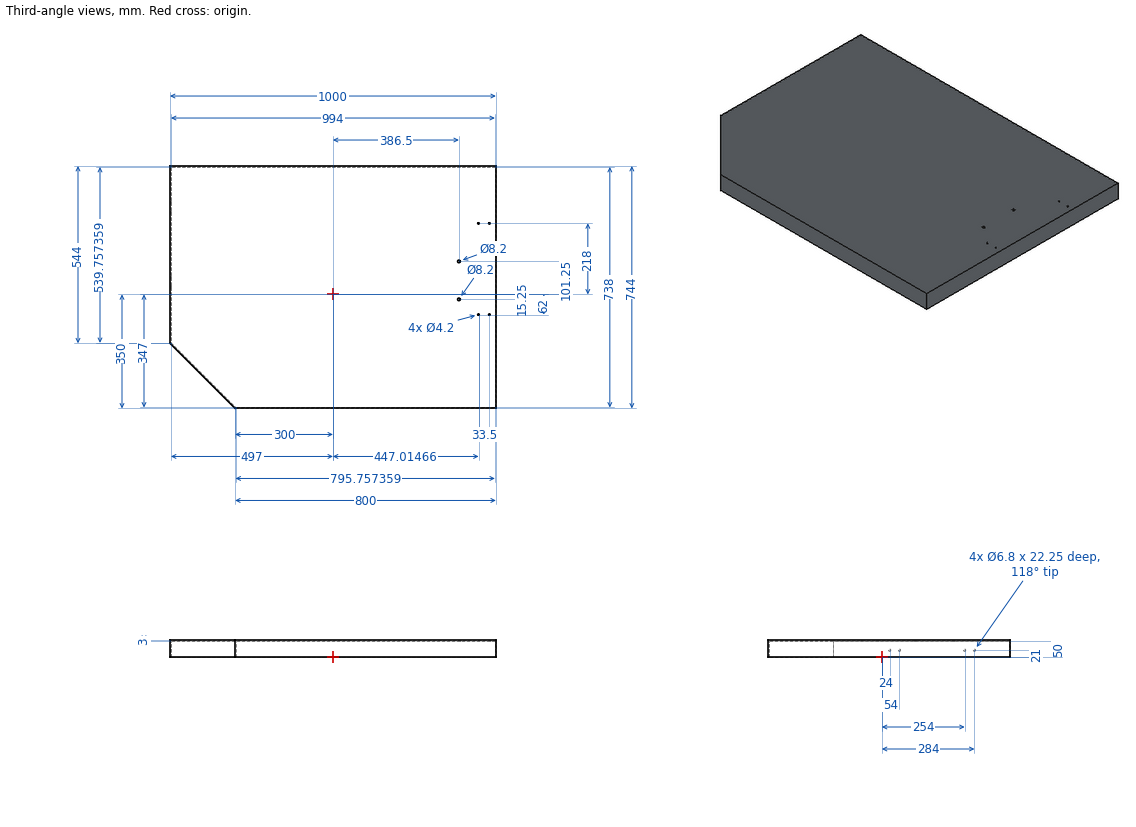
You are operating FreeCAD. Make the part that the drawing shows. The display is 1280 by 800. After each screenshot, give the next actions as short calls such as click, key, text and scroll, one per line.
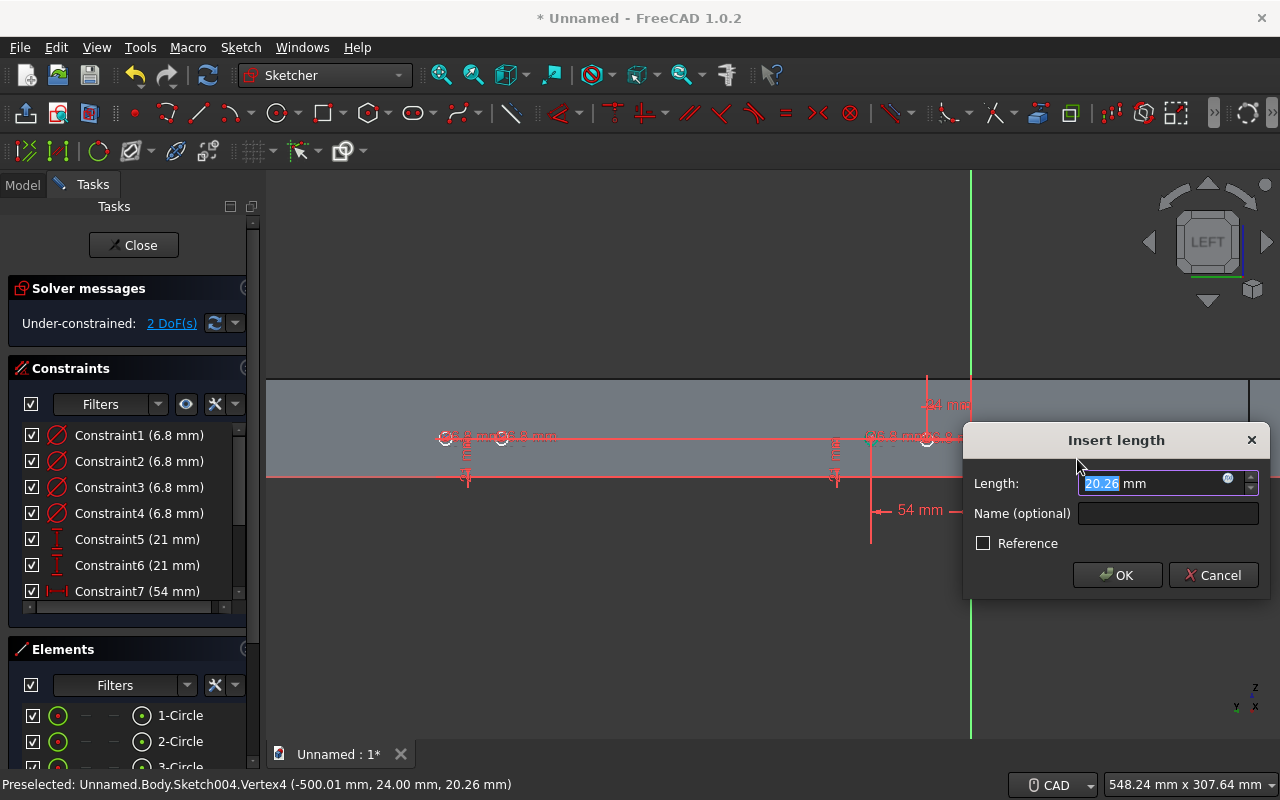
text(21)
key(Return)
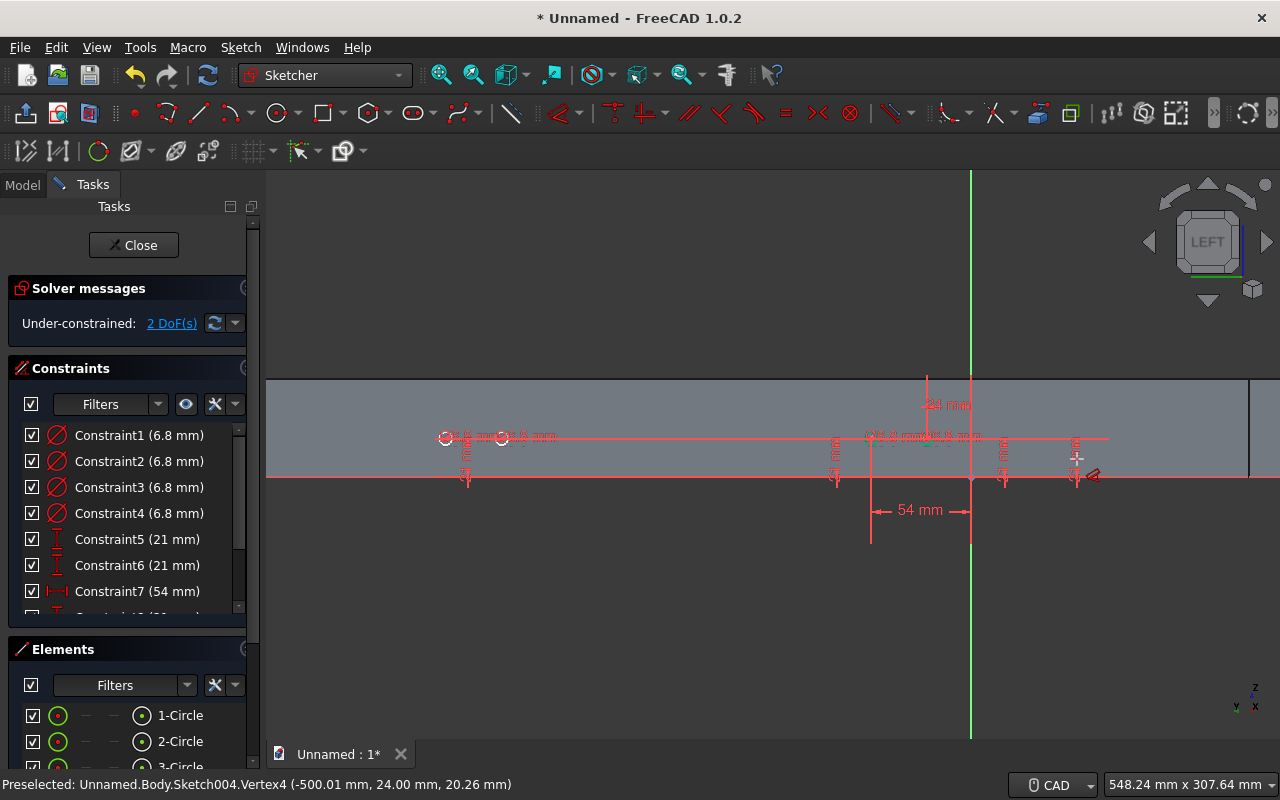
click(446, 439)
click(708, 511)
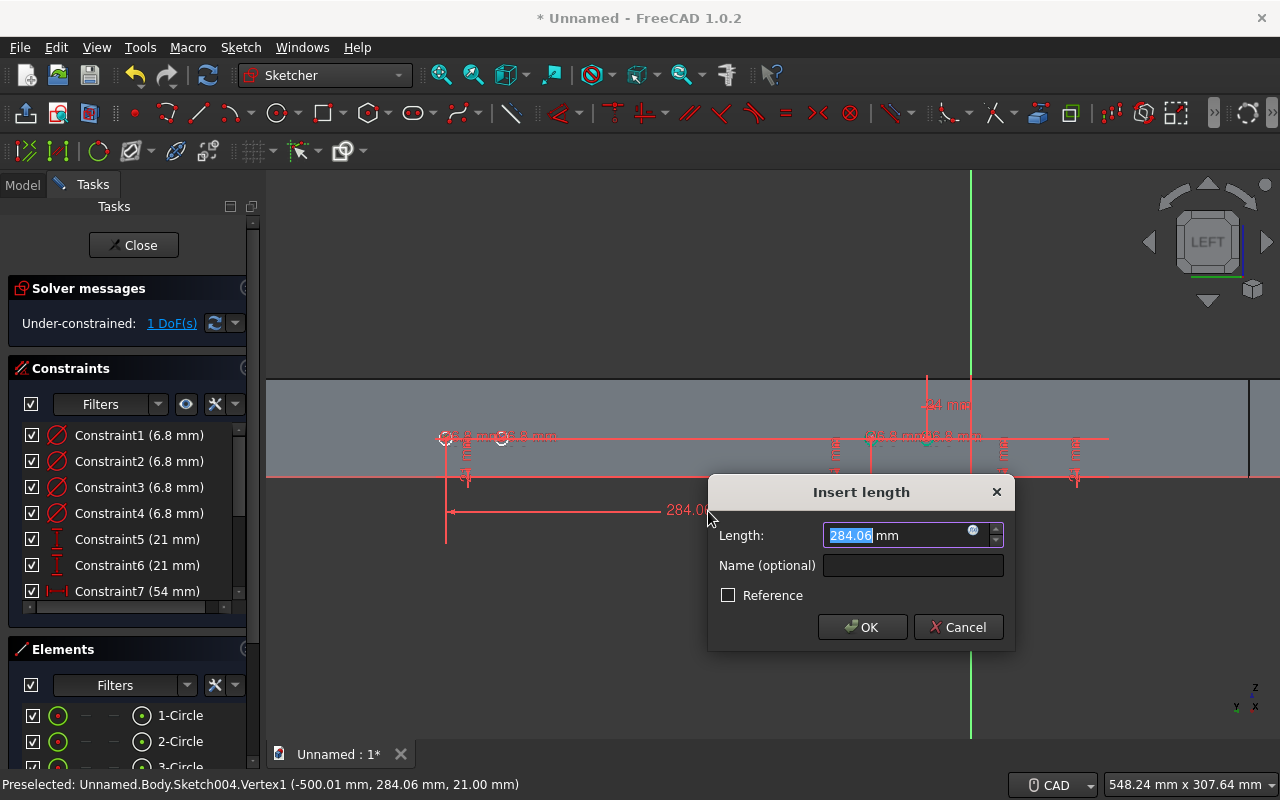
text(284)
key(Return)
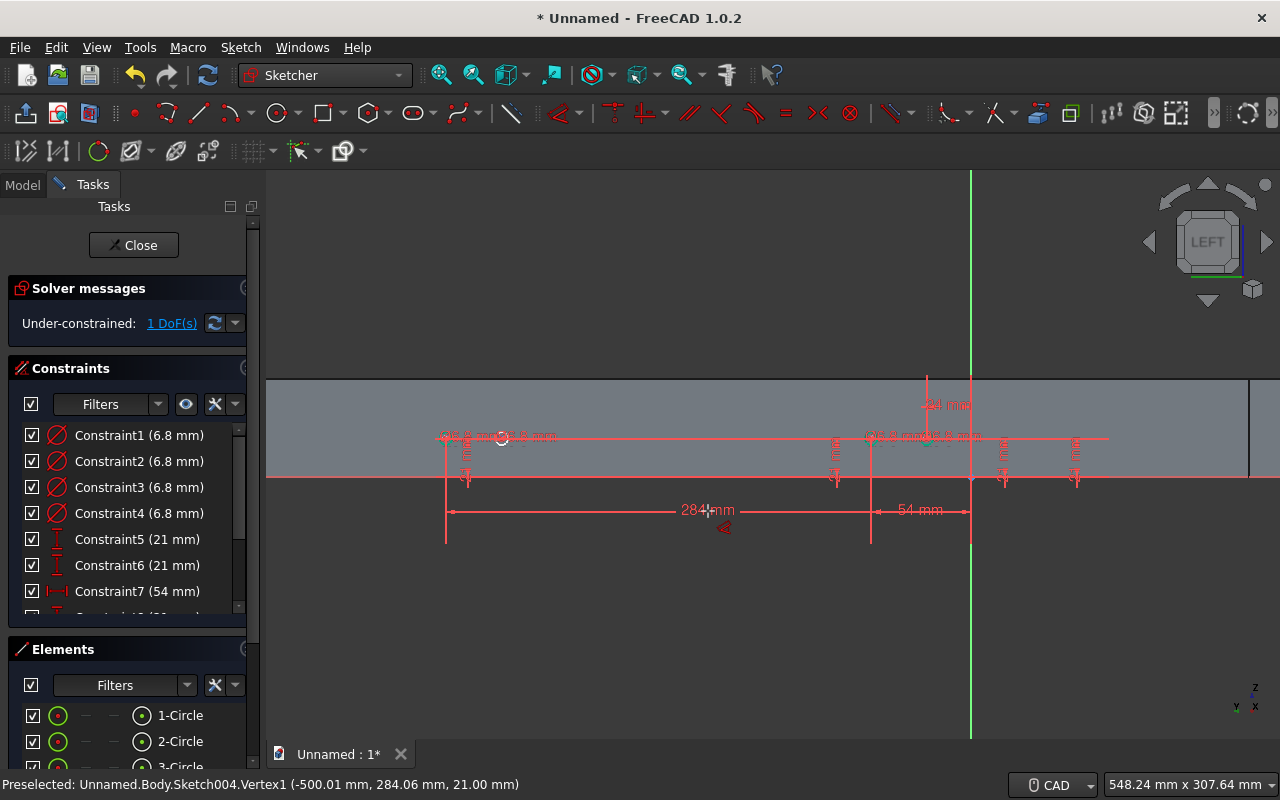
click(502, 439)
click(628, 511)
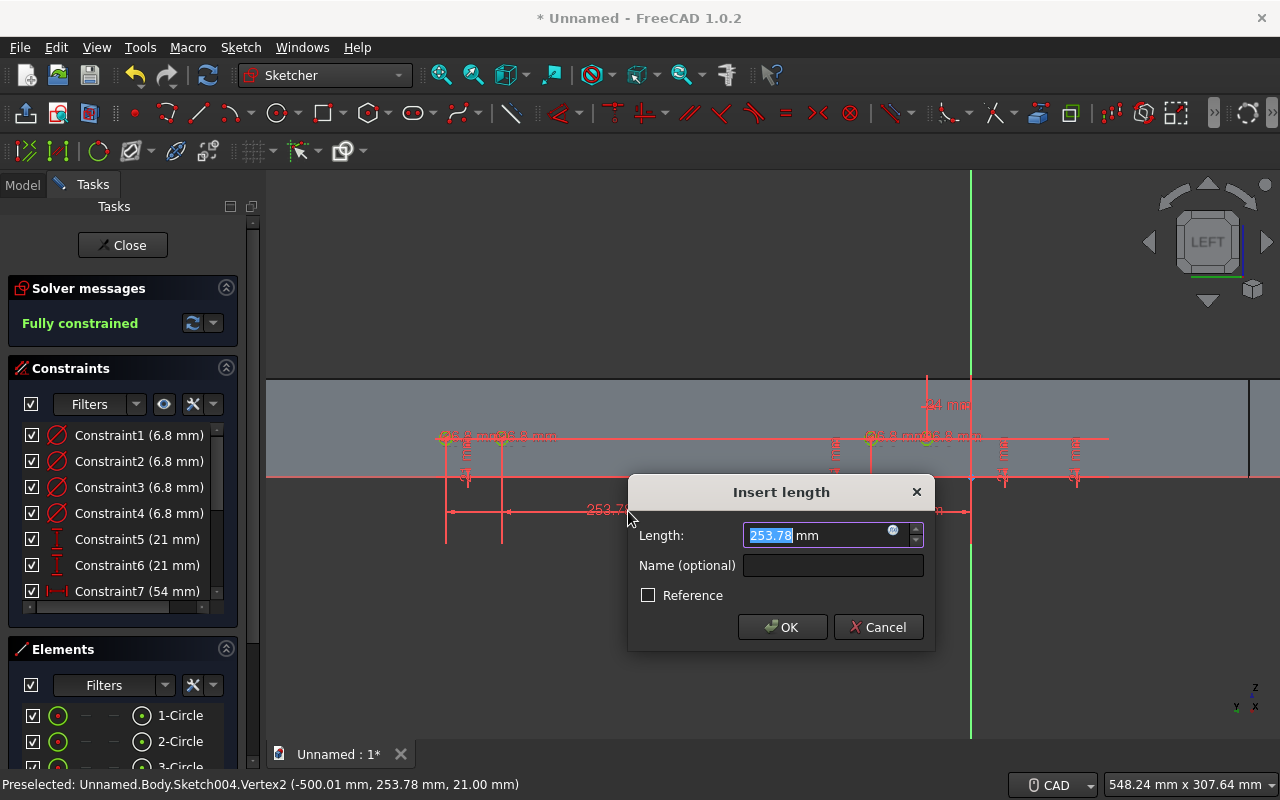
text(254)
key(Return)
key(Escape)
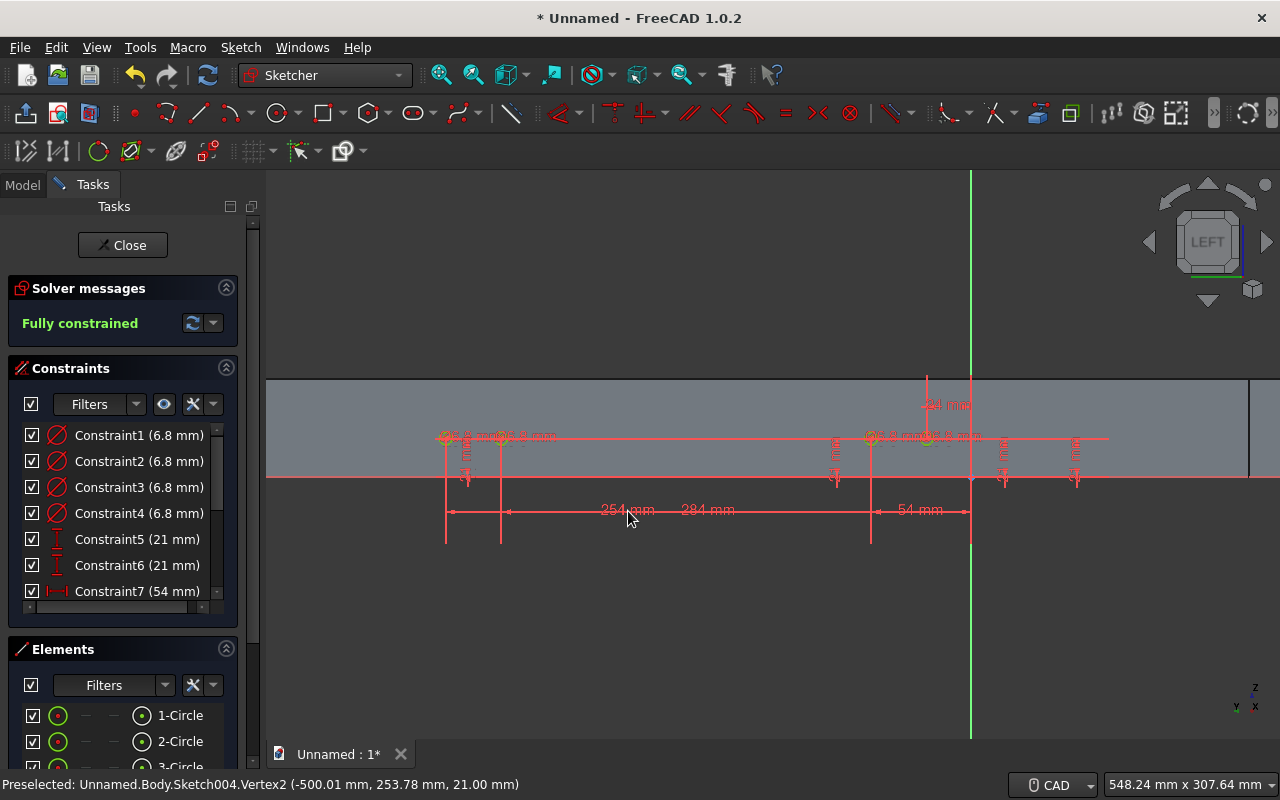
click(123, 245)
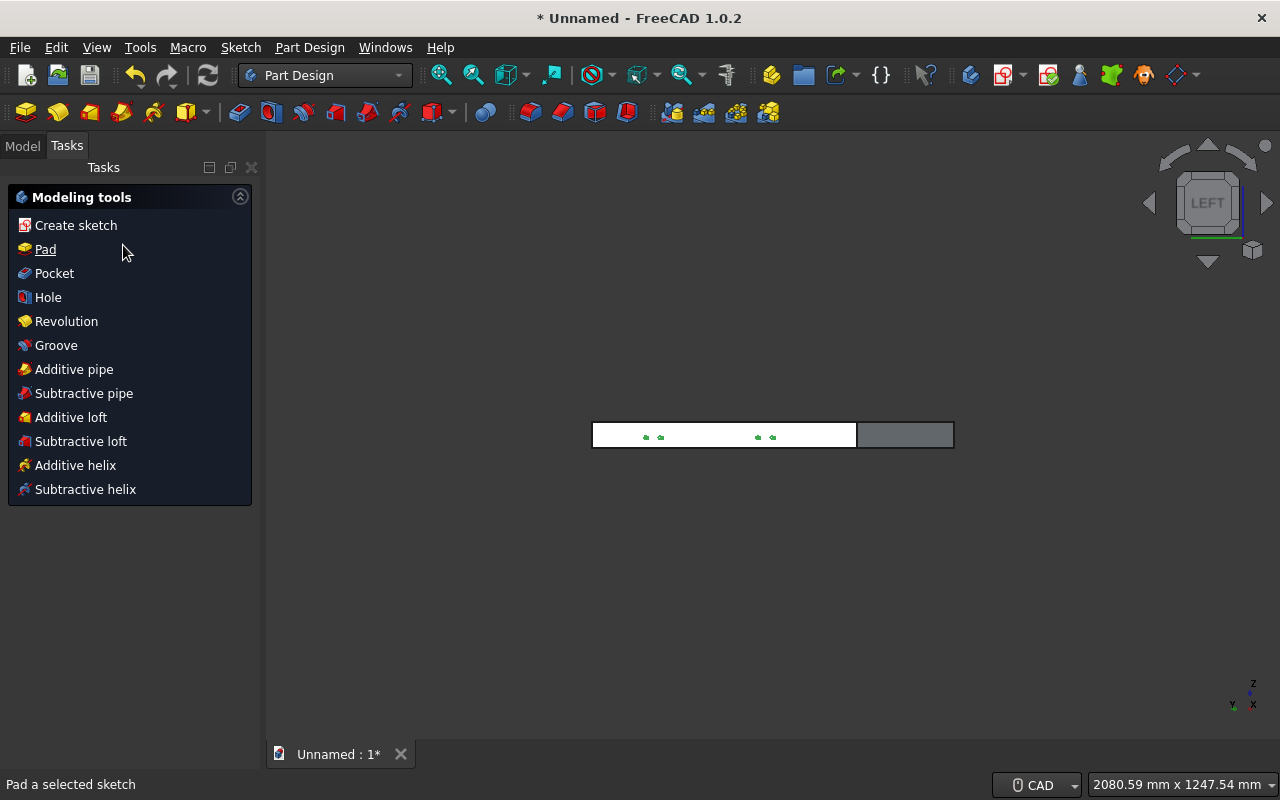
click(272, 112)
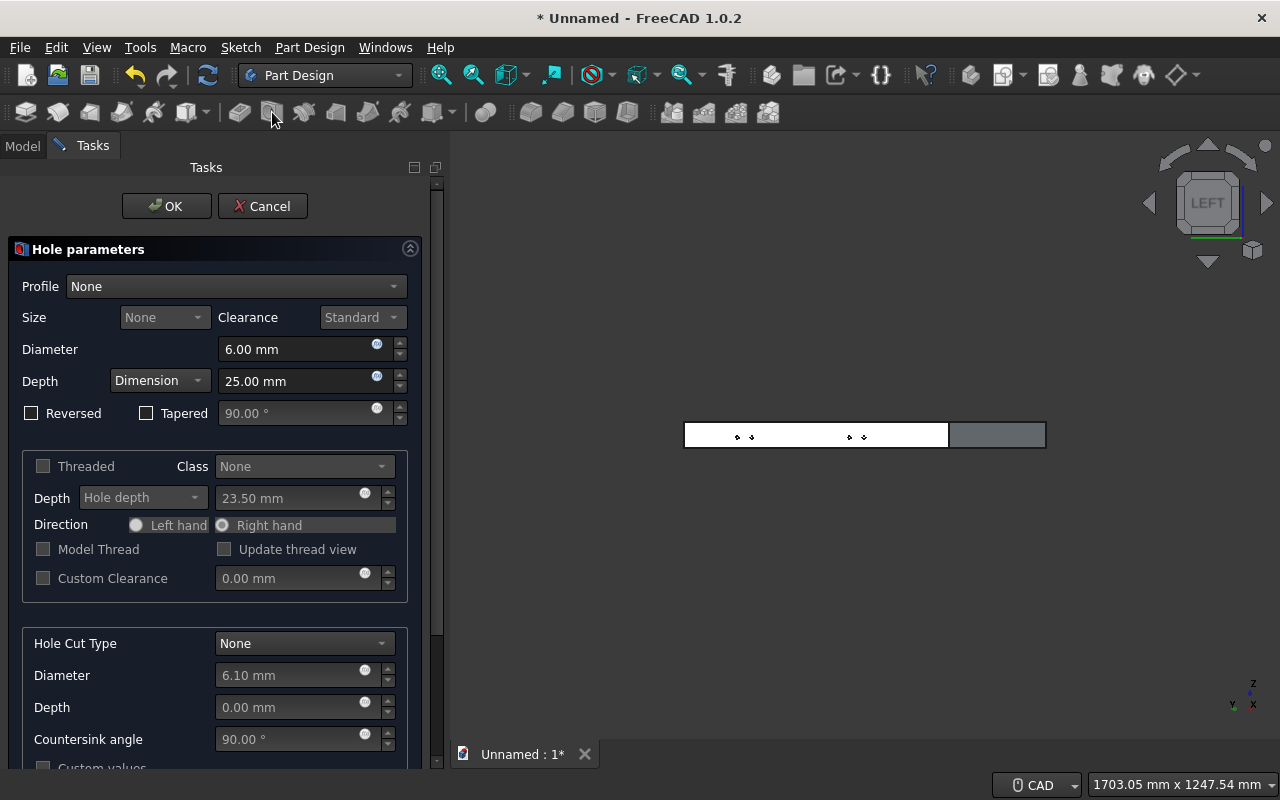
triple_click(305, 349)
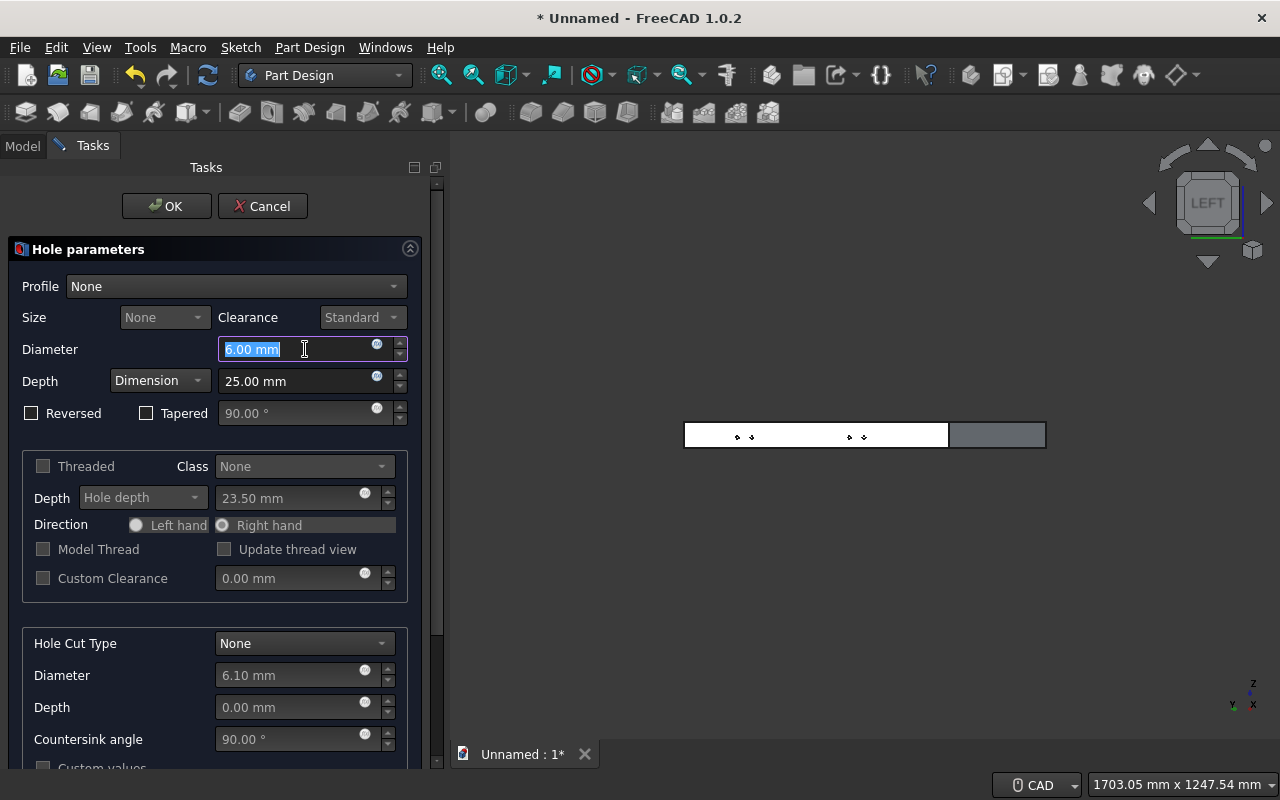
text(6.8)
key(Tab)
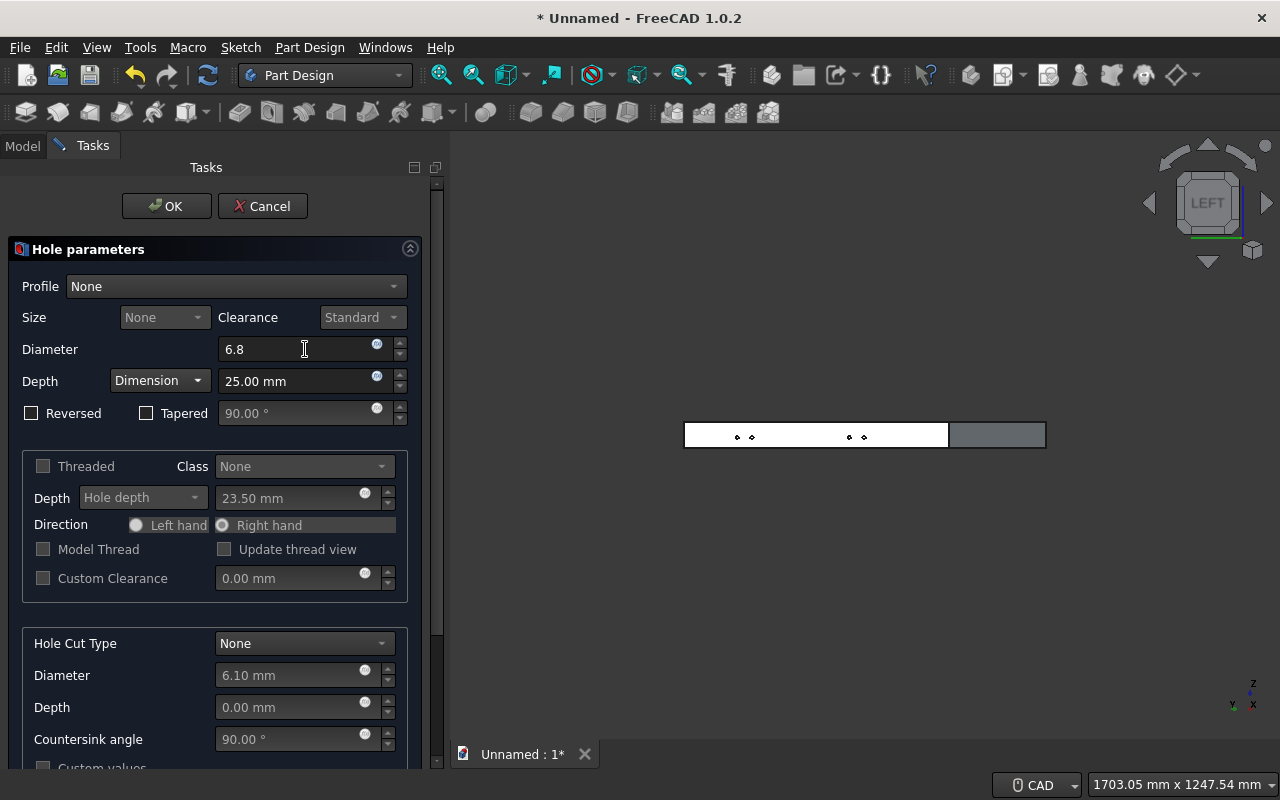
triple_click(305, 381)